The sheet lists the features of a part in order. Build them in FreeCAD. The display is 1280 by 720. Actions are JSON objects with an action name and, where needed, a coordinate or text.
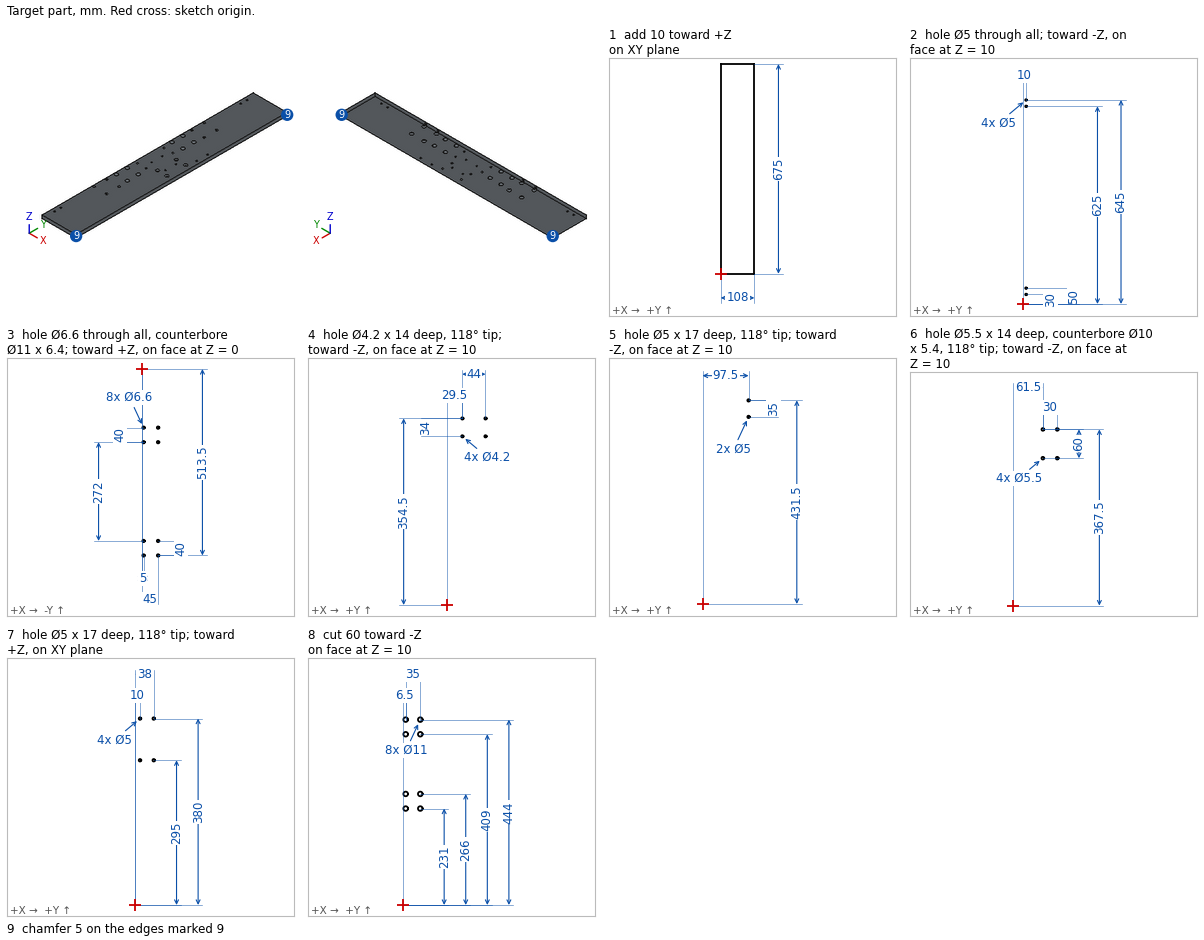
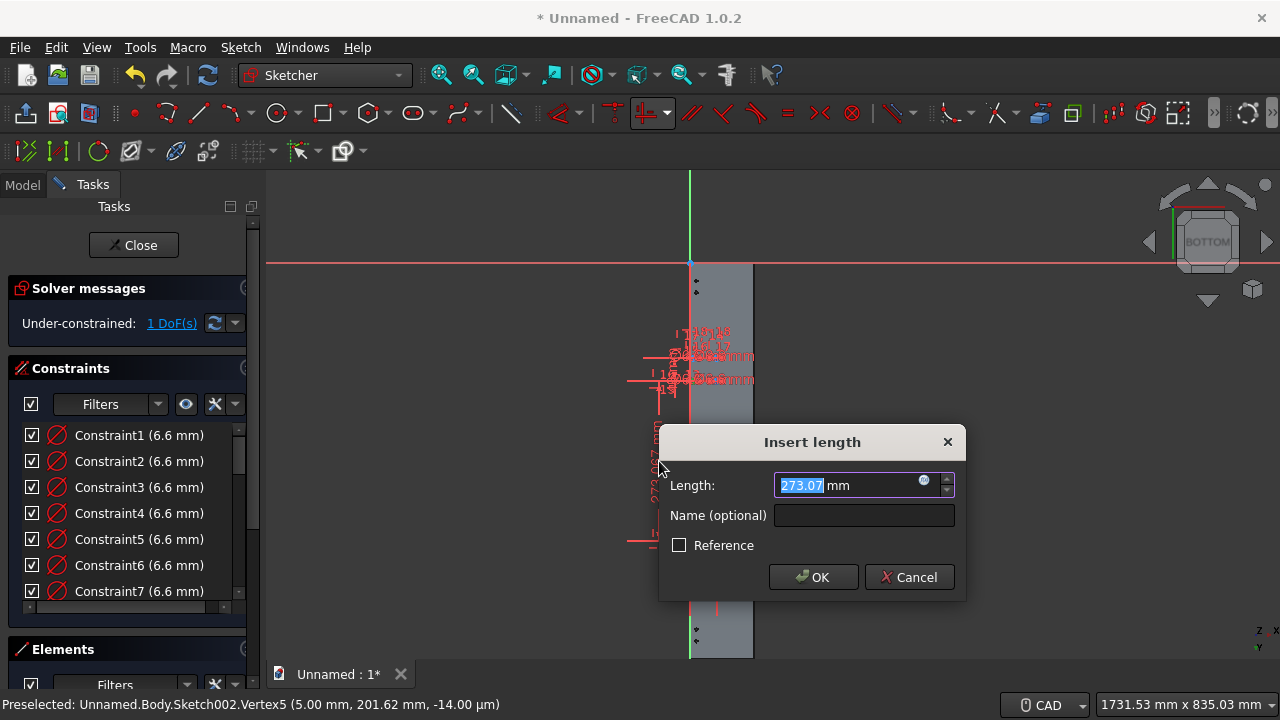
{"action": "type", "text": "272"}
{"action": "key", "text": "Return"}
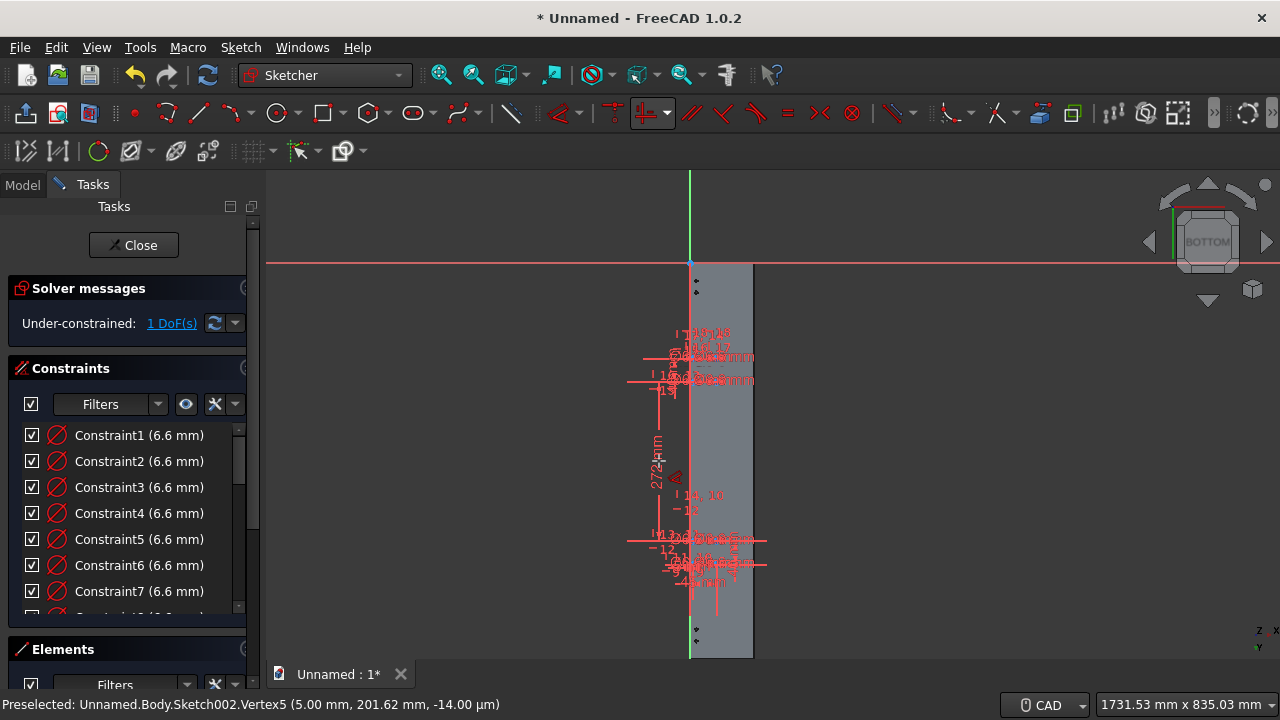
{"action": "left_click", "coordinate": [717, 565]}
{"action": "left_click", "coordinate": [656, 414]}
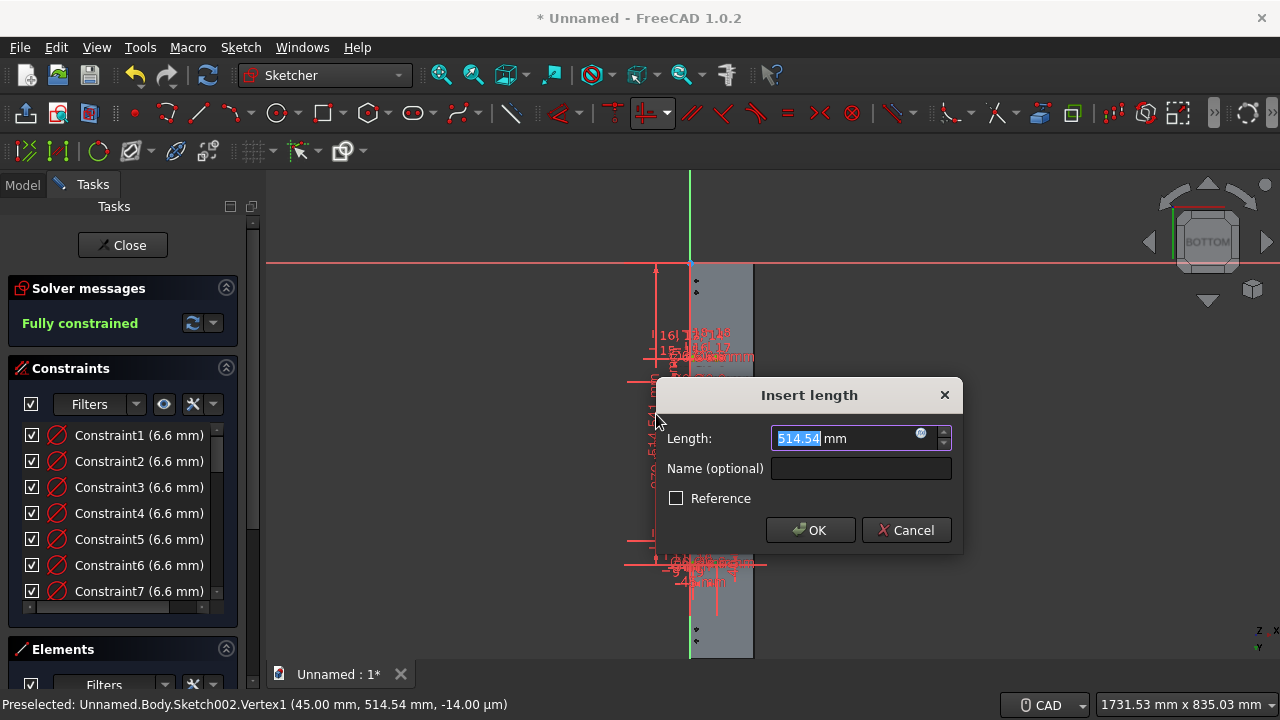
{"action": "type", "text": "513.5"}
{"action": "key", "text": "Return"}
{"action": "key", "text": "Escape"}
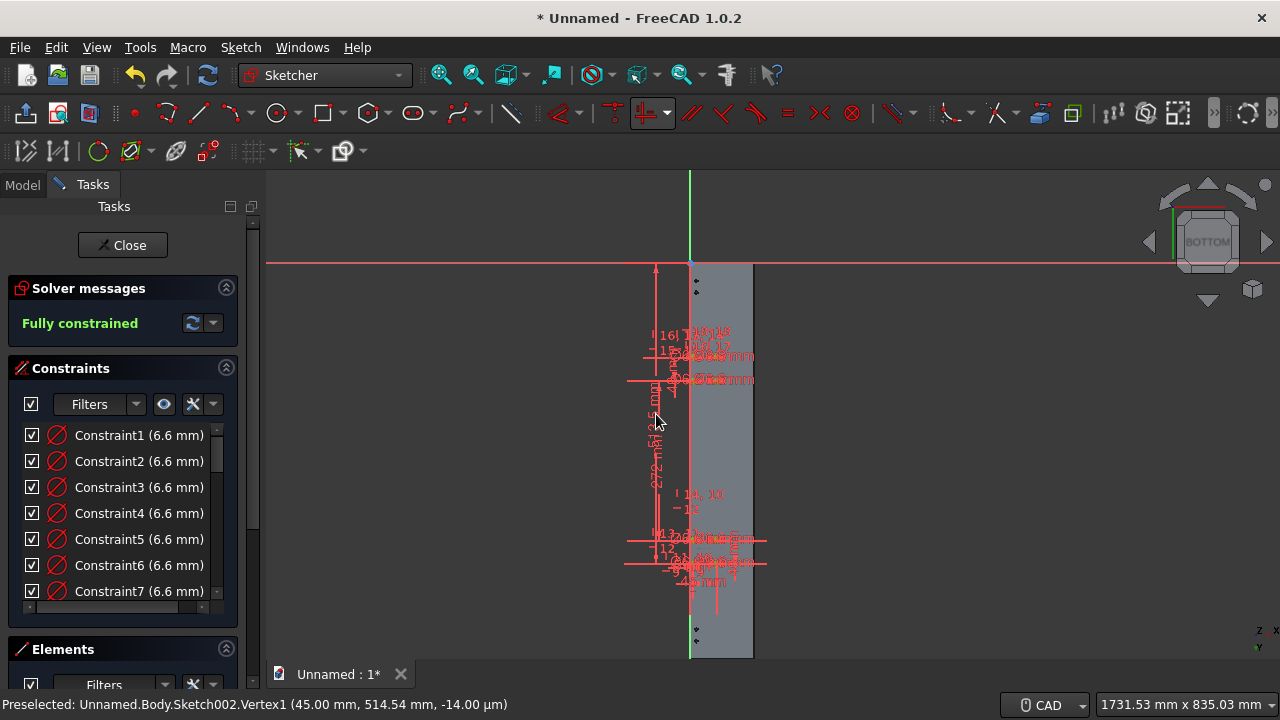
{"action": "left_click", "coordinate": [123, 245]}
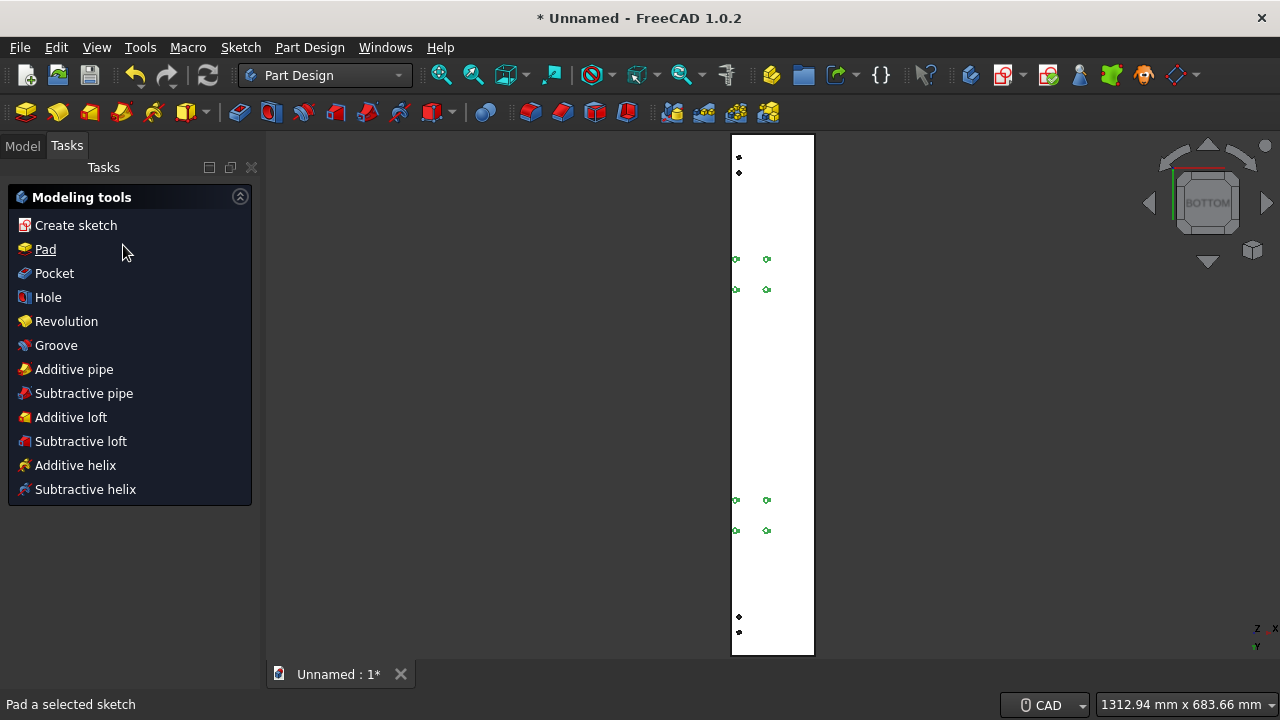
{"action": "left_click", "coordinate": [272, 112]}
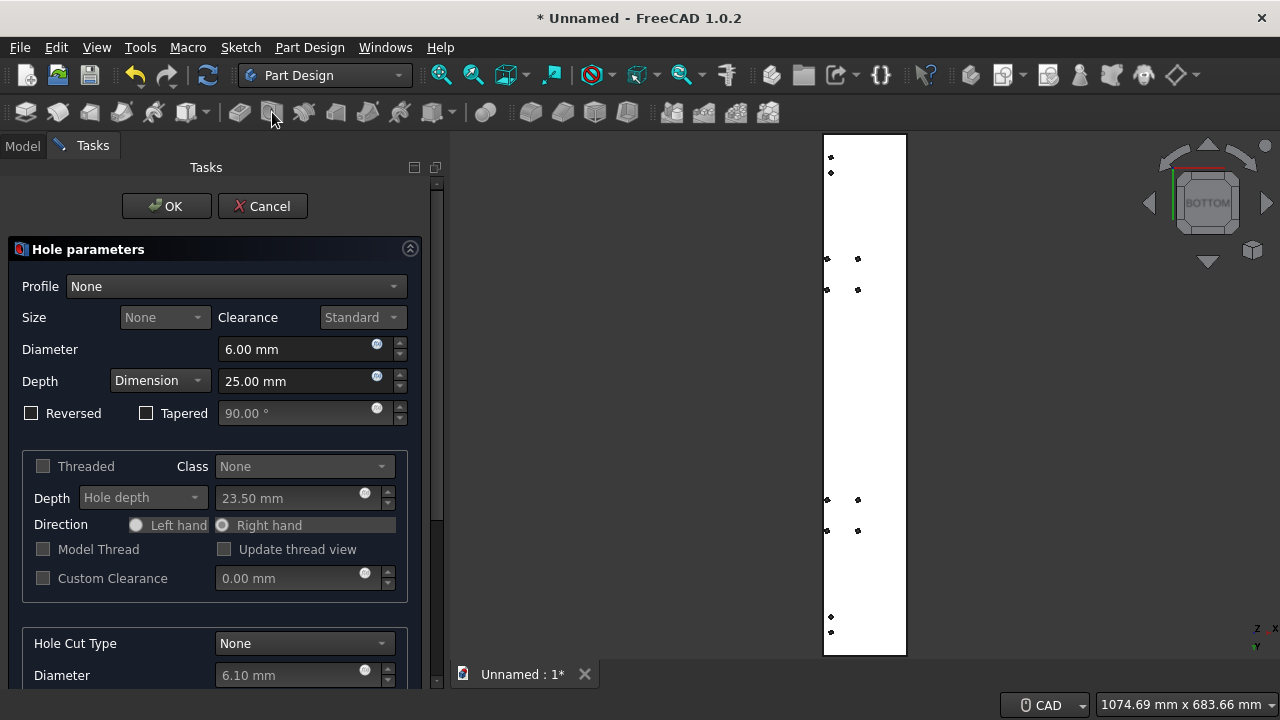
{"action": "triple_click", "coordinate": [305, 349]}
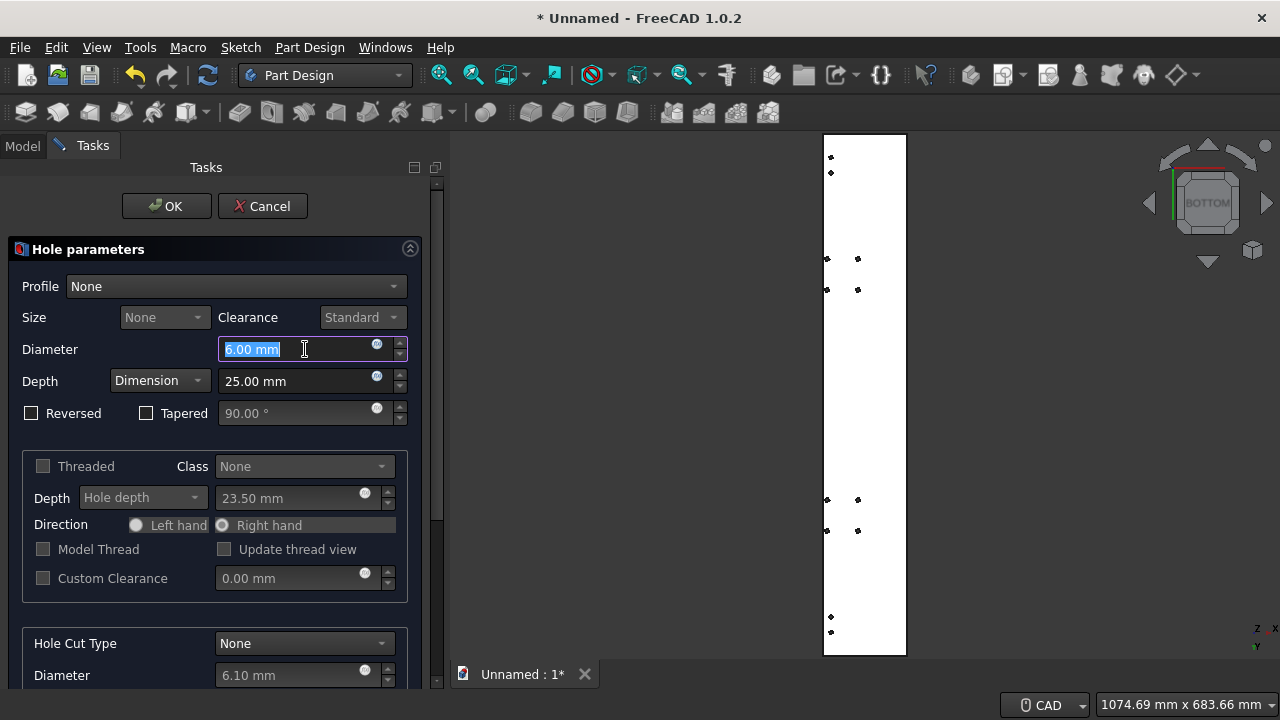
{"action": "type", "text": "6.6"}
{"action": "key", "text": "Tab"}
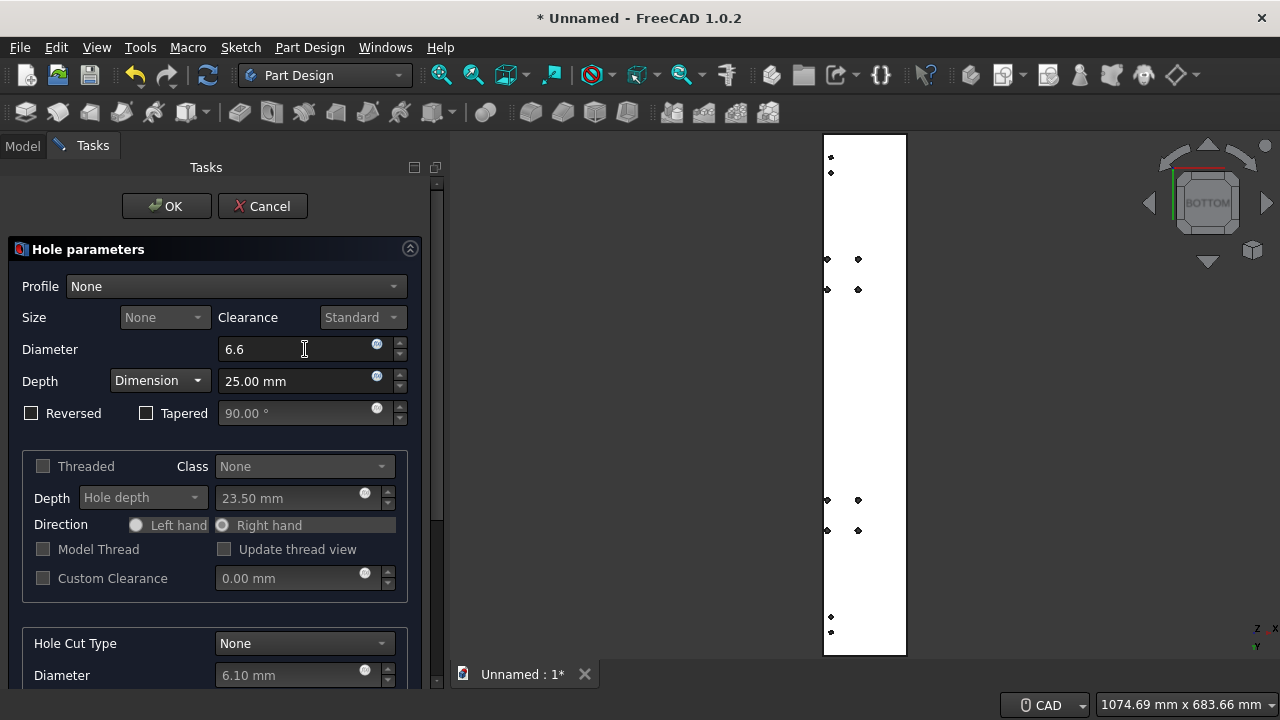
{"action": "left_click", "coordinate": [161, 380]}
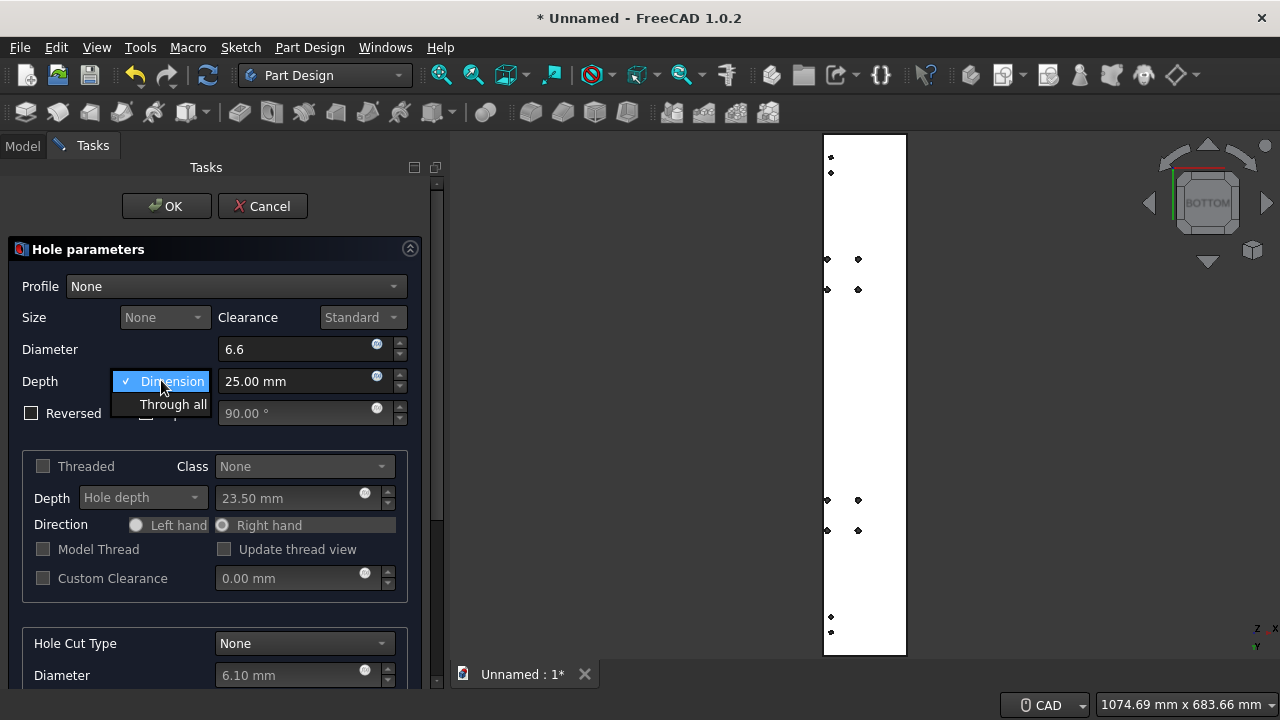
{"action": "left_click", "coordinate": [160, 404]}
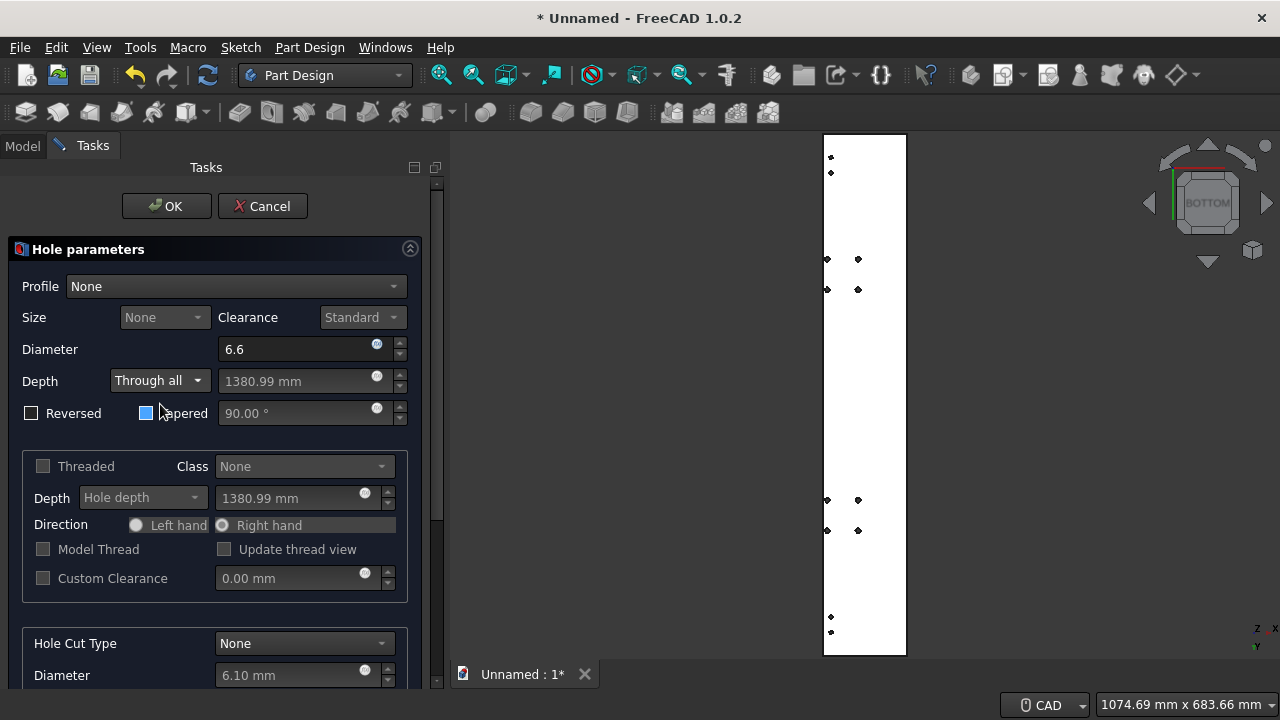
{"action": "left_click", "coordinate": [306, 644]}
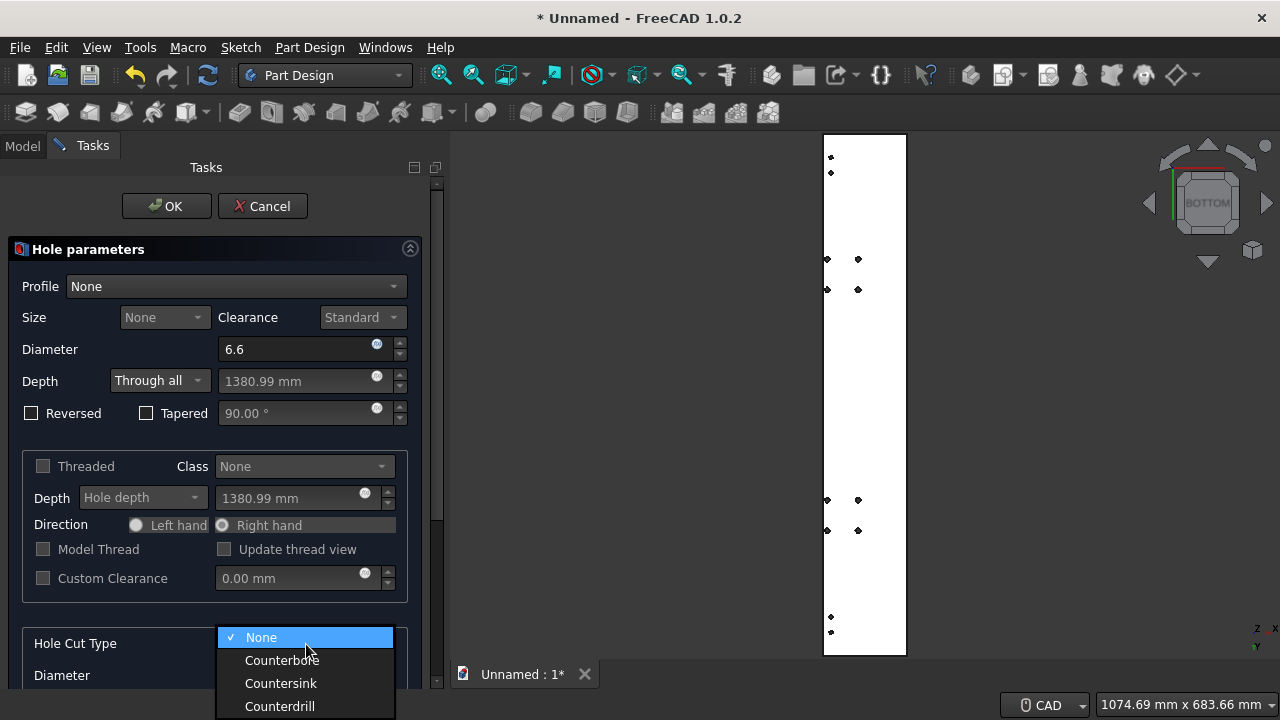
{"action": "left_click", "coordinate": [304, 660]}